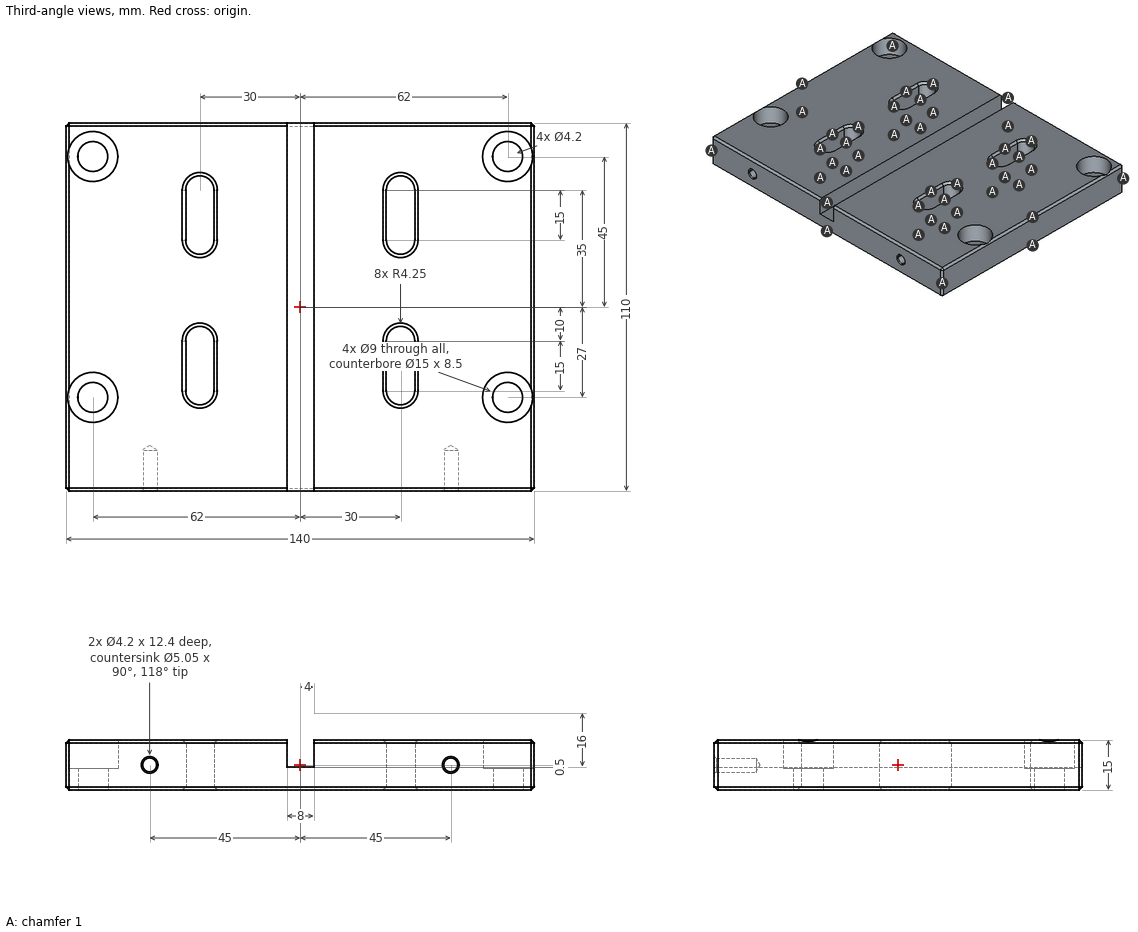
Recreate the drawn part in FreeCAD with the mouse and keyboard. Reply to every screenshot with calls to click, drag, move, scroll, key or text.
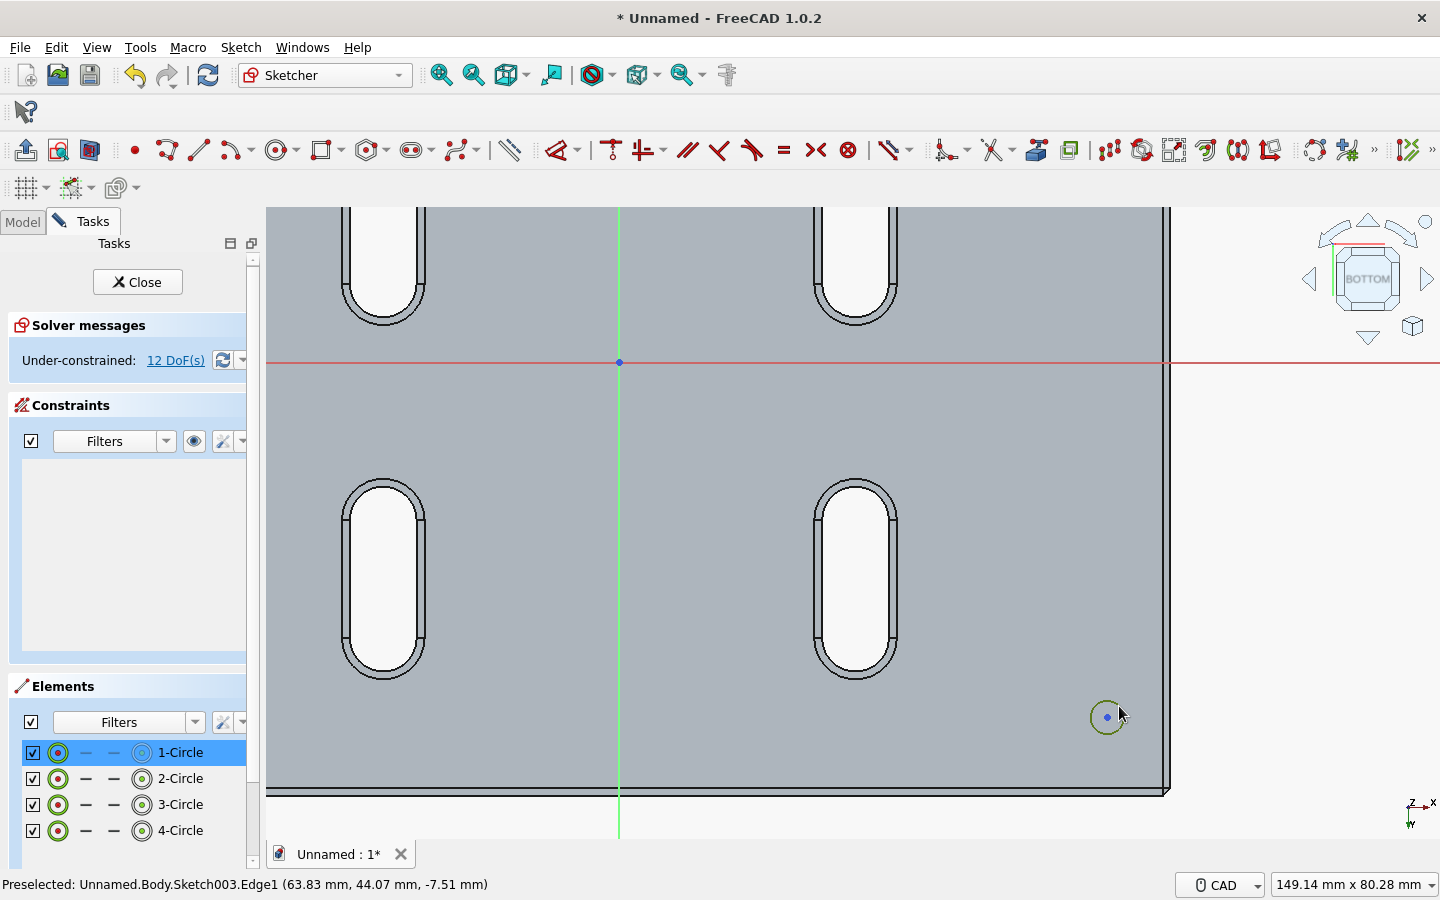
scroll(1120, 705, down, 2)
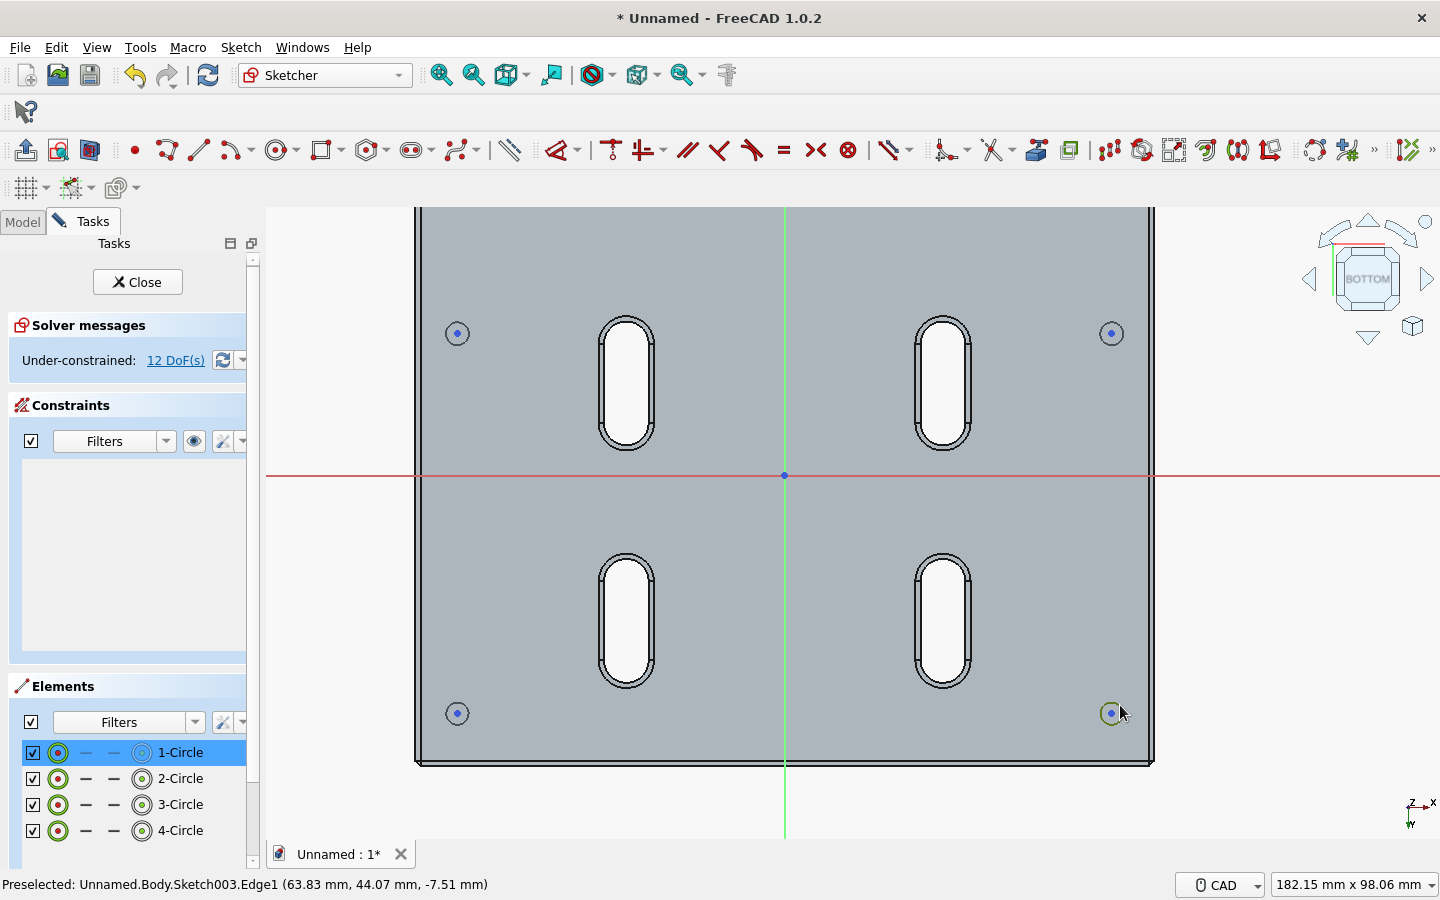
click(1120, 326)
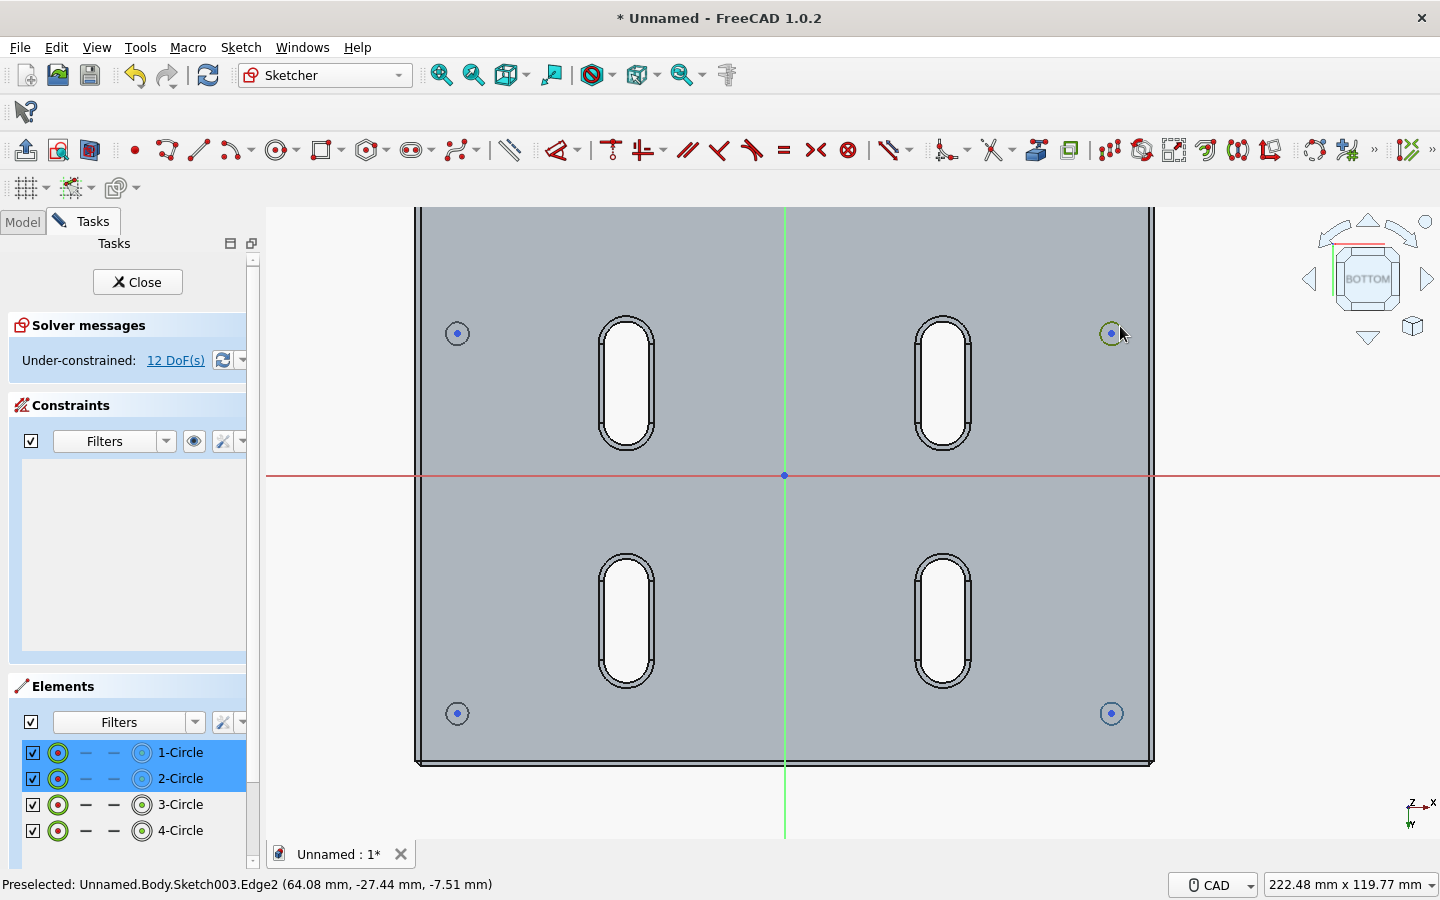
click(465, 326)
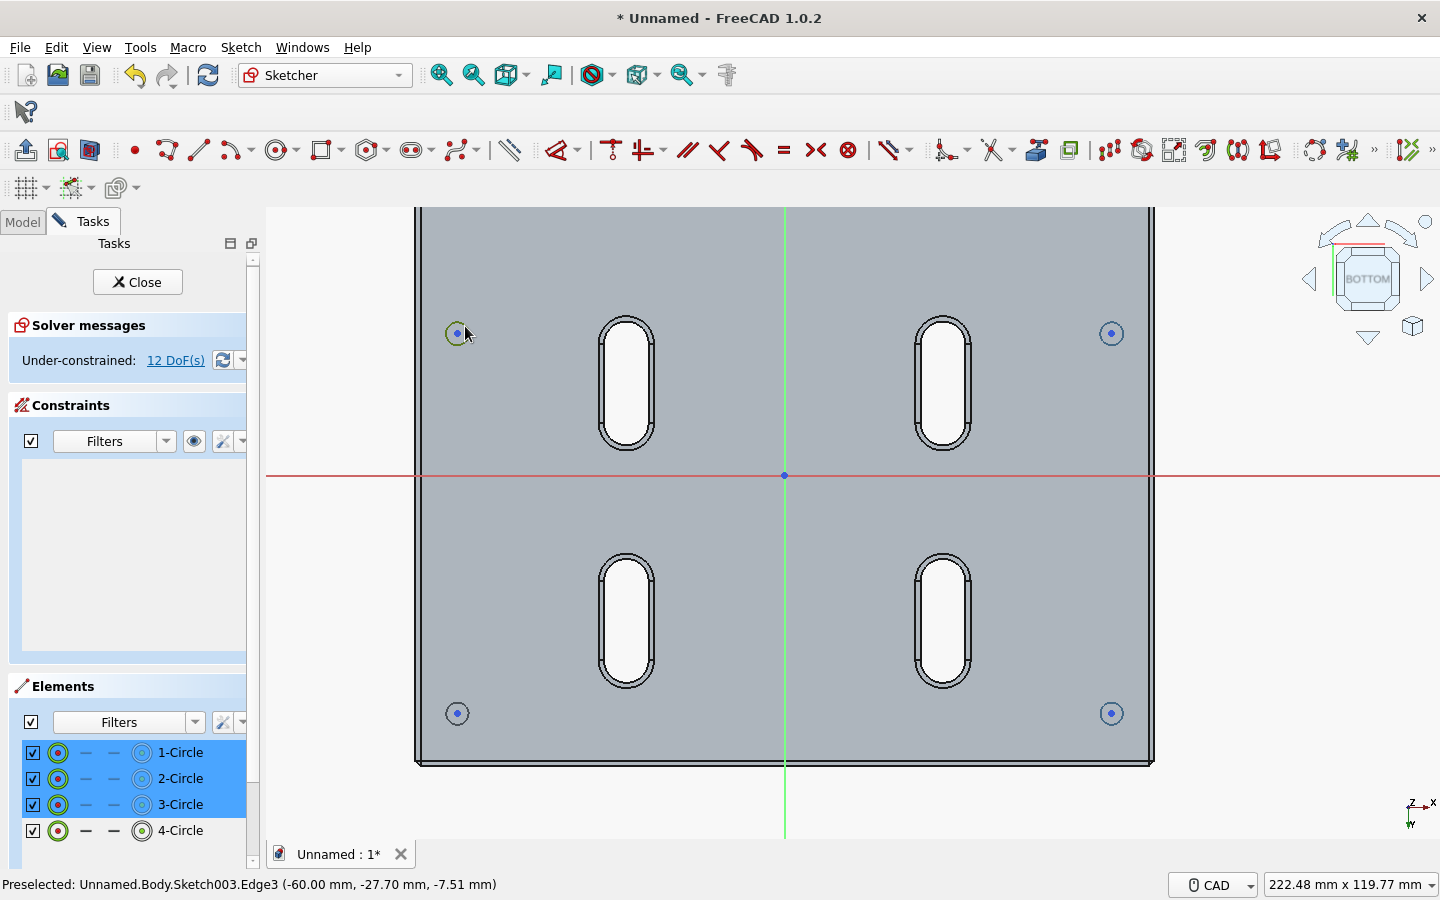
scroll(465, 706, up, 2)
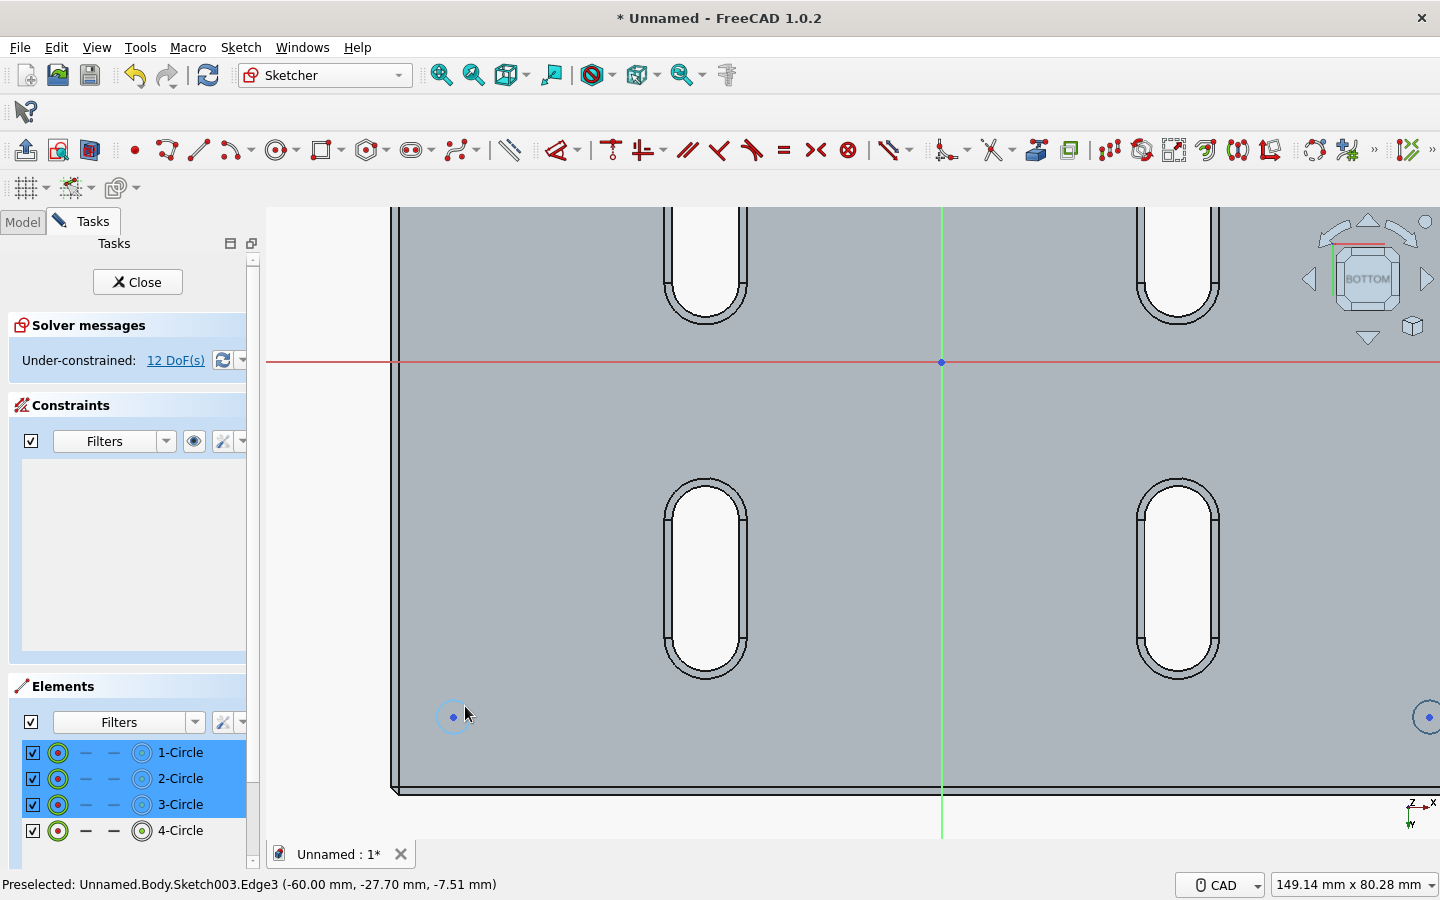
click(465, 705)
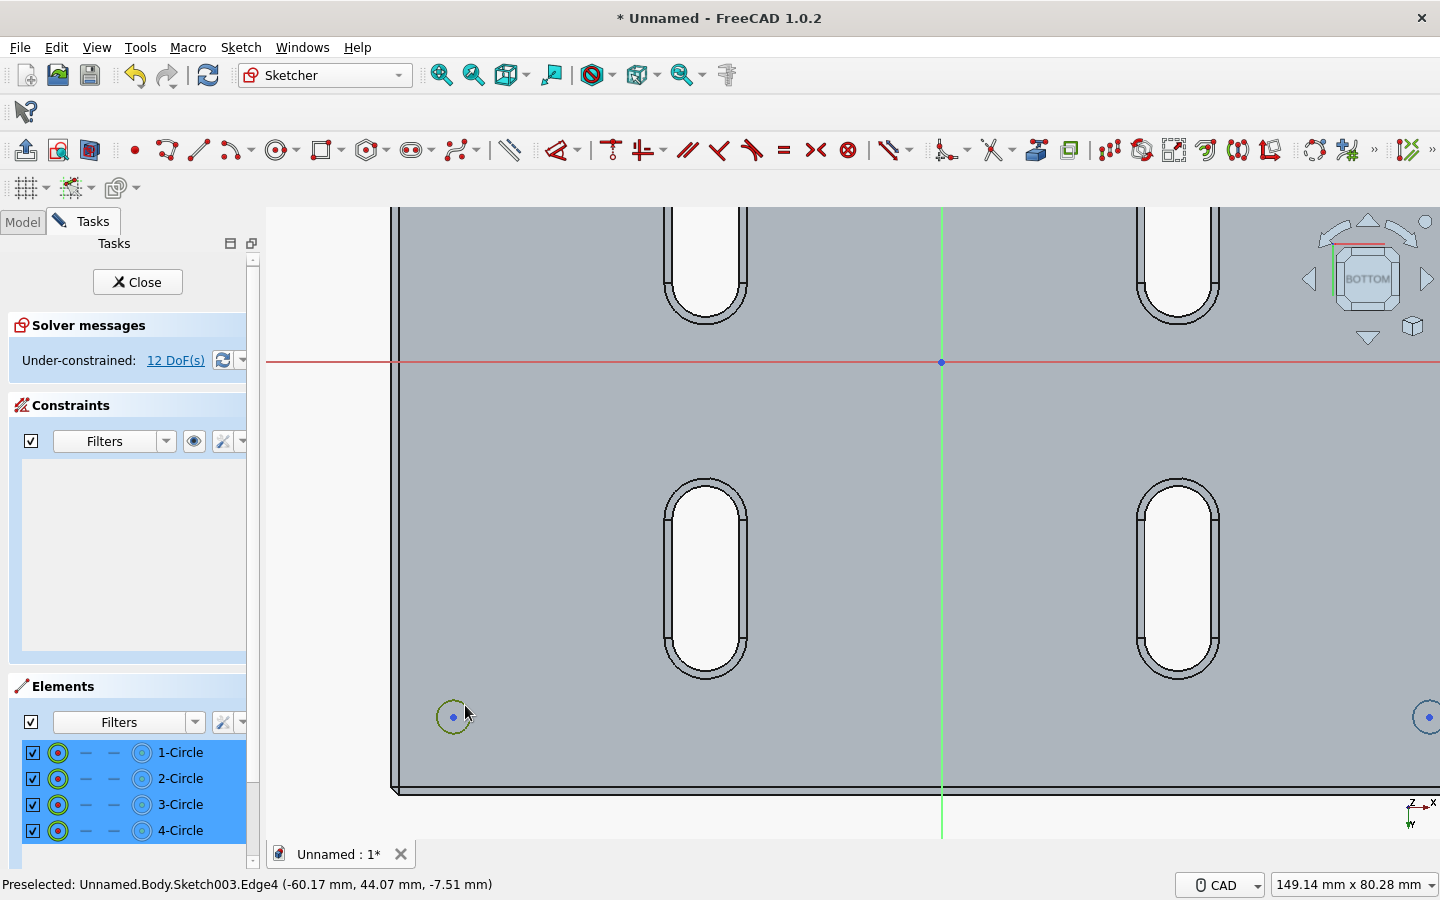
key(e)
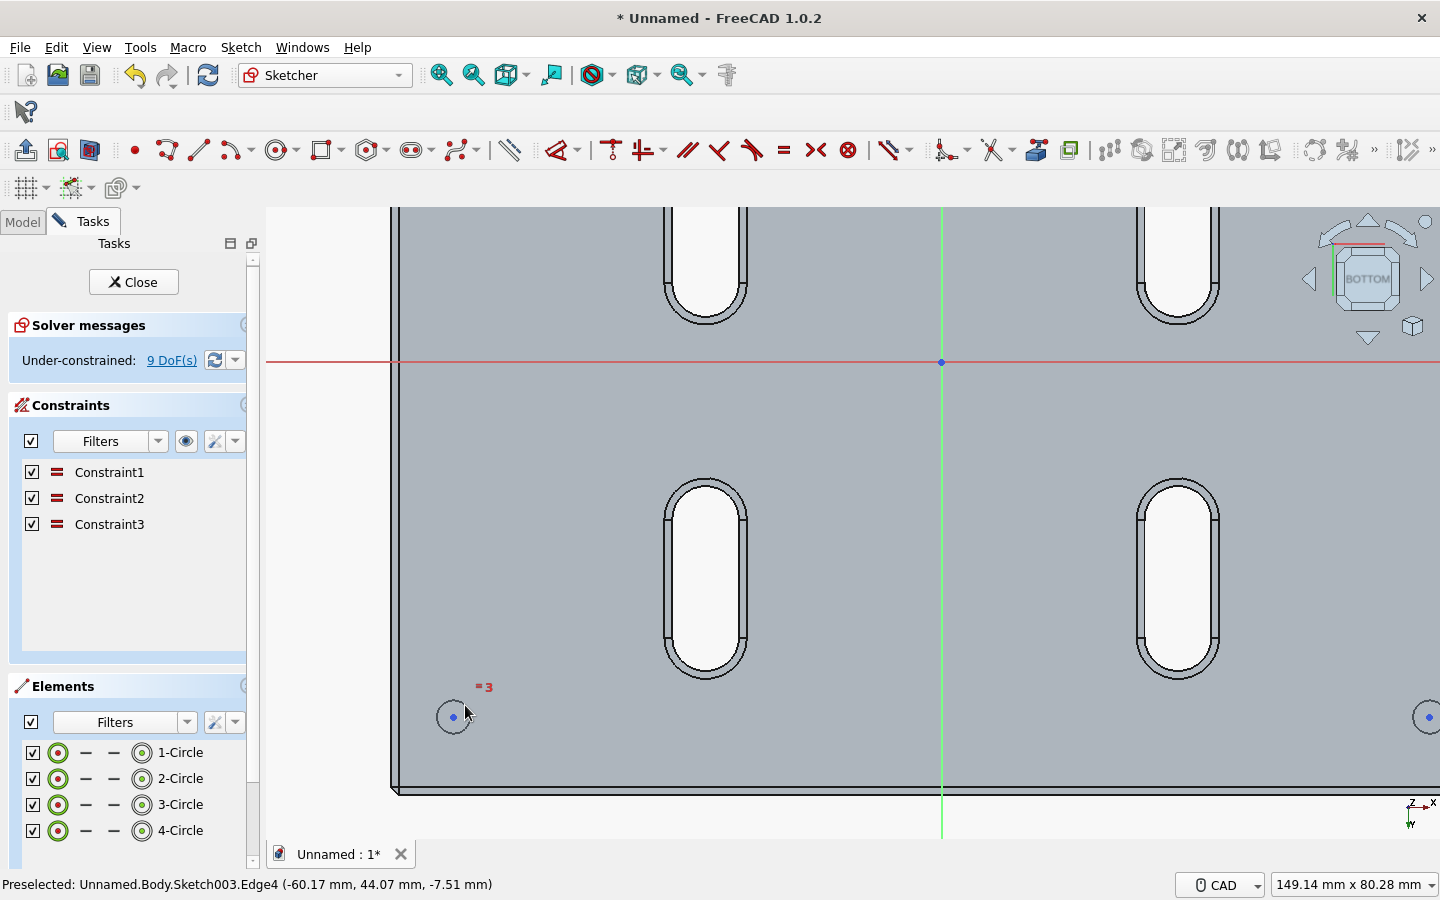
scroll(465, 706, down, 2)